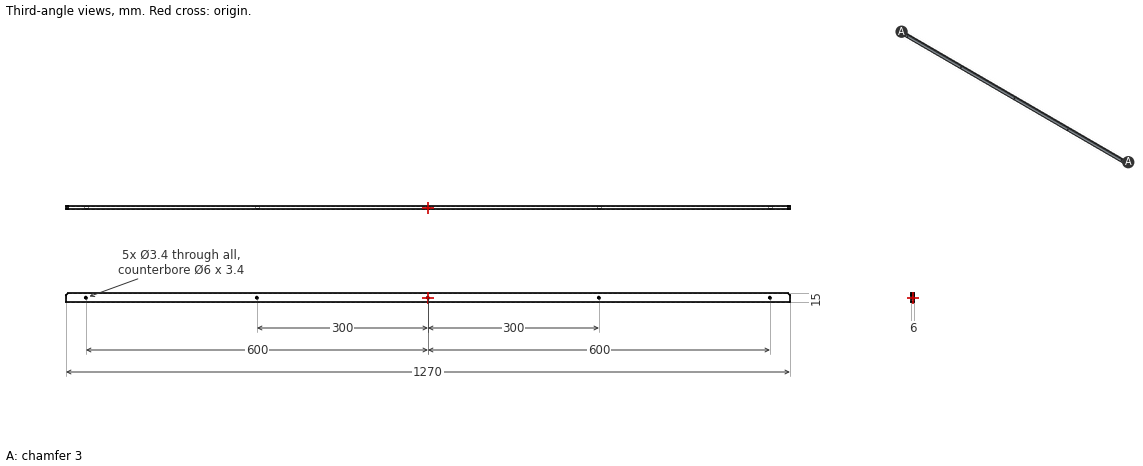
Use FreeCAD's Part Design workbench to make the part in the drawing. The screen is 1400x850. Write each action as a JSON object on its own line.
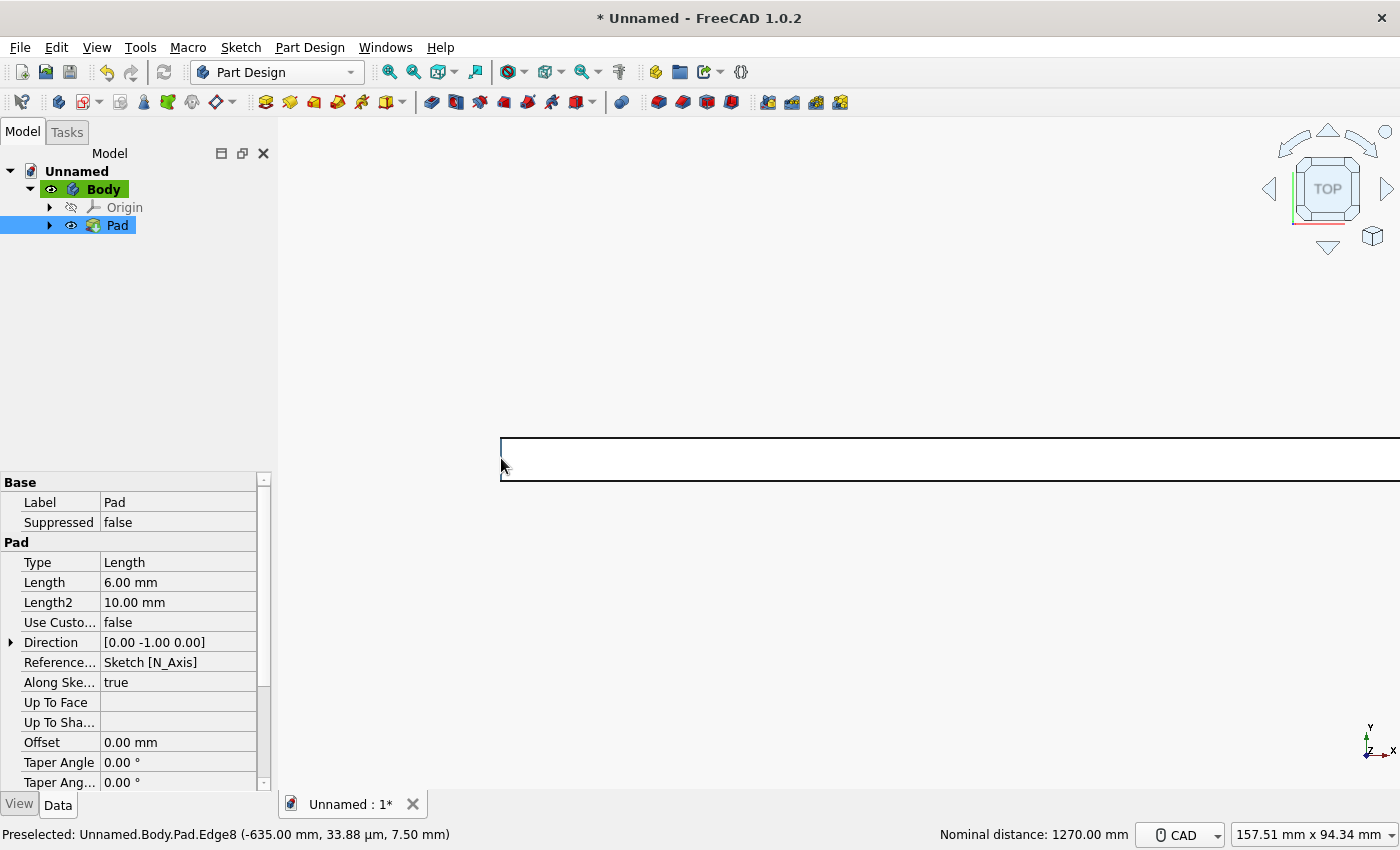
{"action": "left_click", "coordinate": [684, 102]}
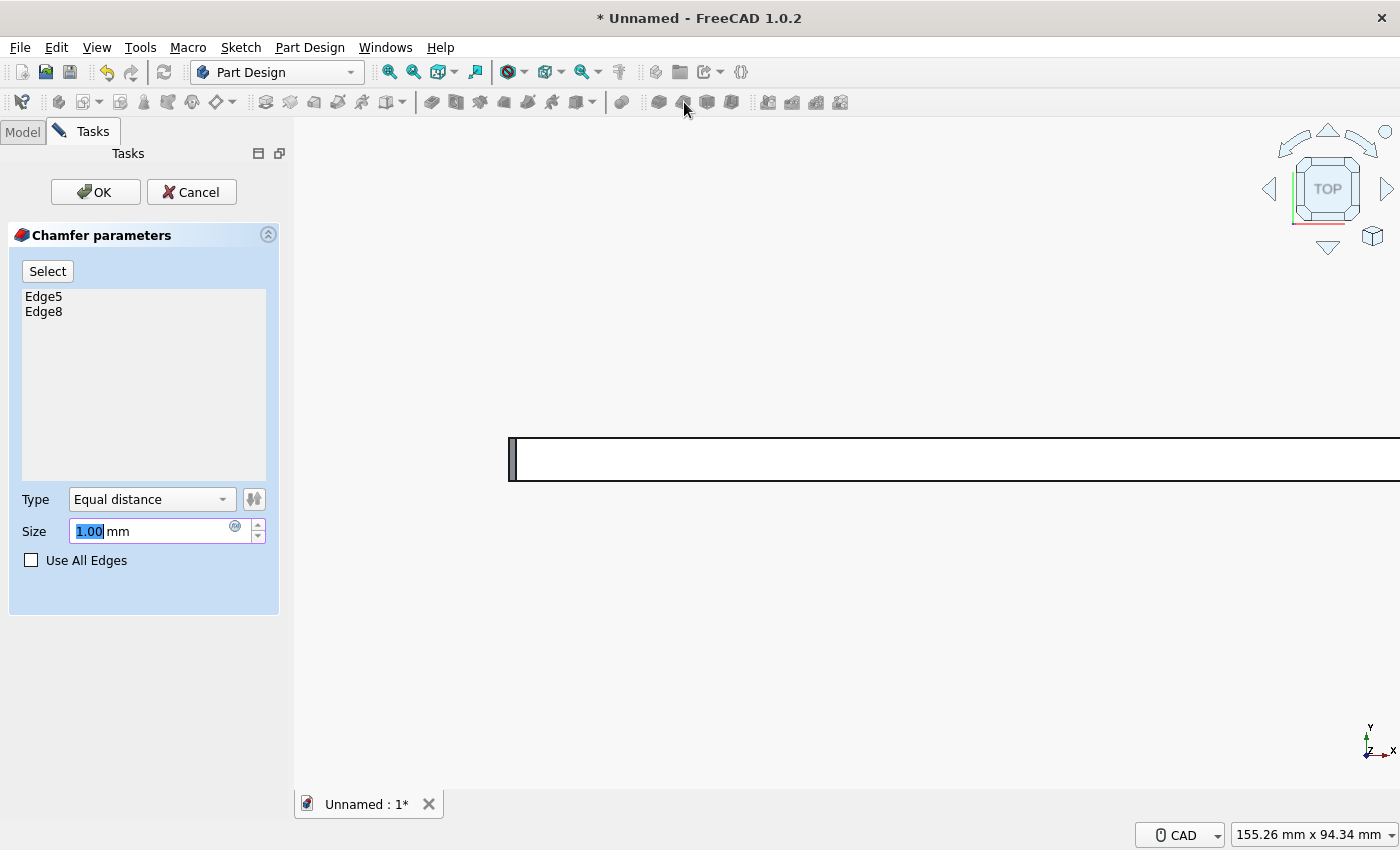
{"action": "type", "text": "3"}
{"action": "key", "text": "Tab"}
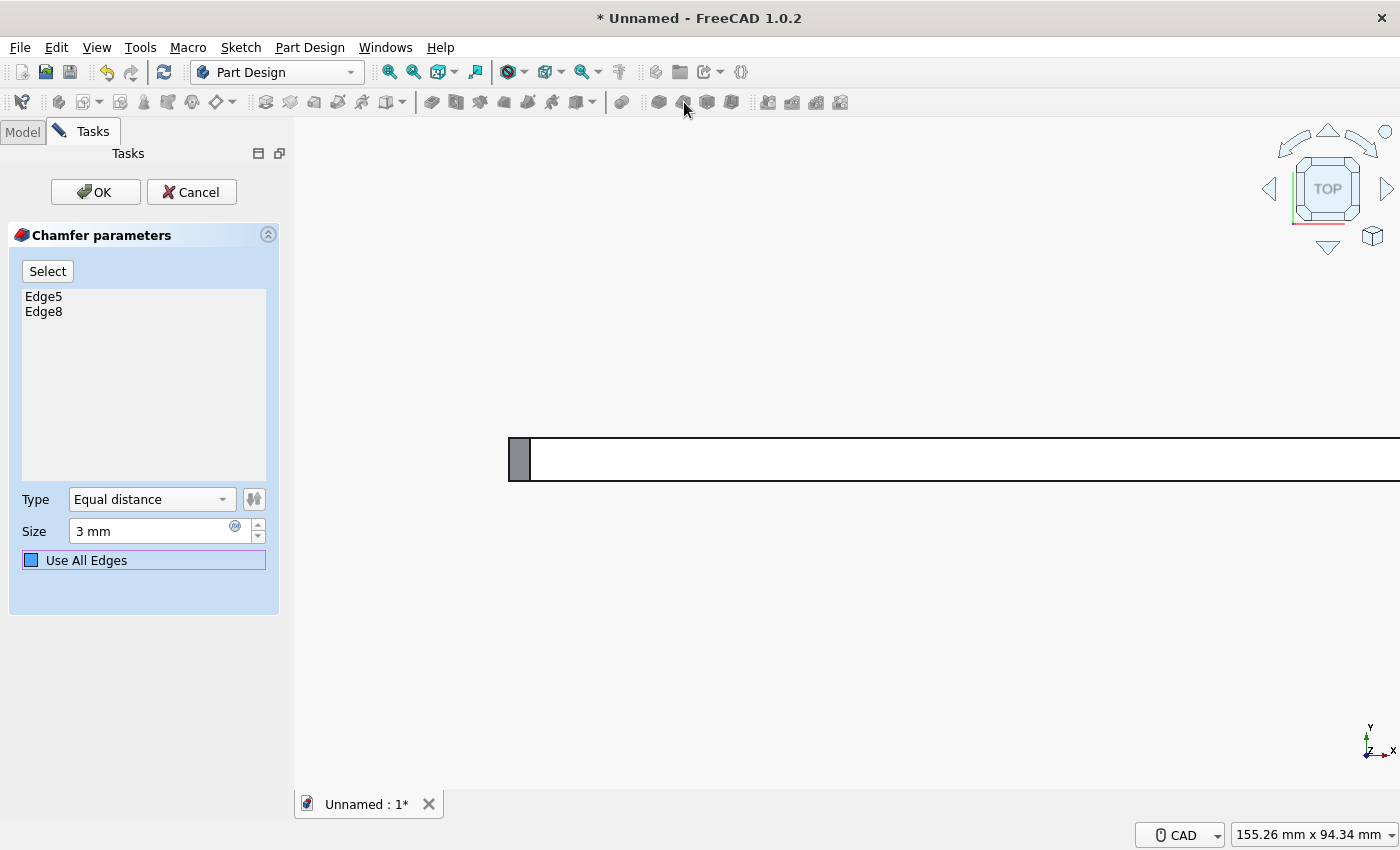
{"action": "left_click", "coordinate": [96, 192]}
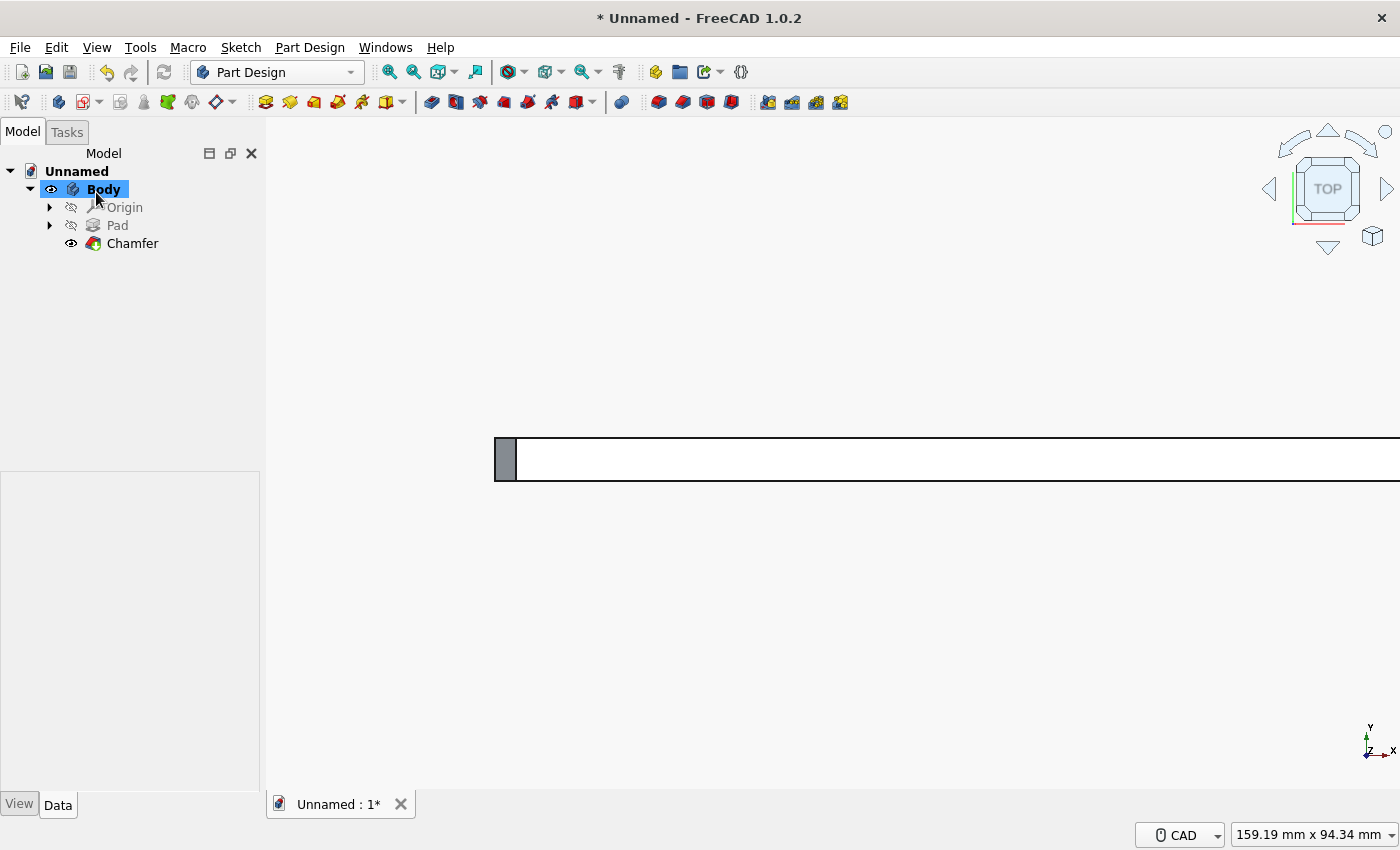
{"action": "left_click", "coordinate": [390, 72]}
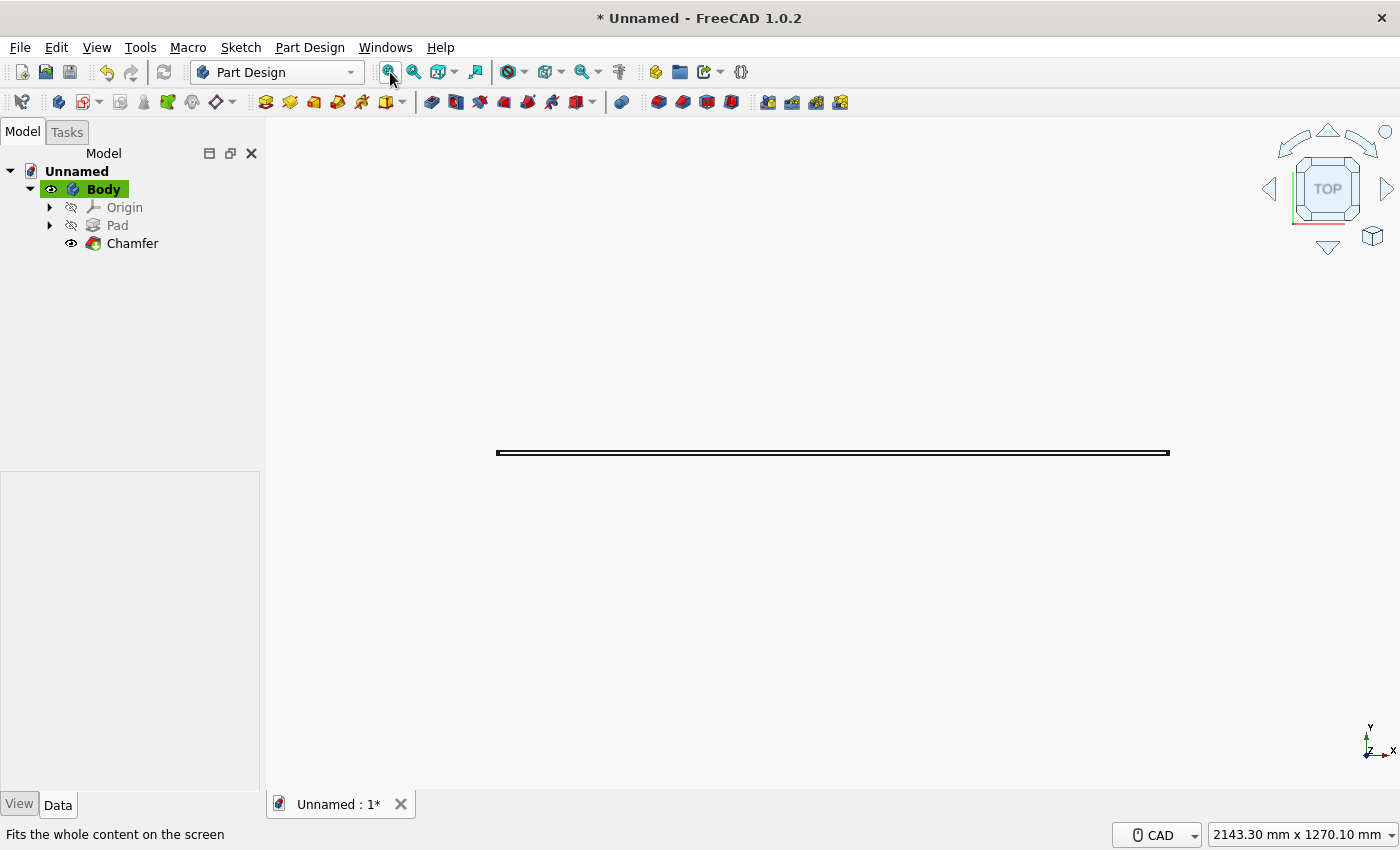
{"action": "key", "text": "4"}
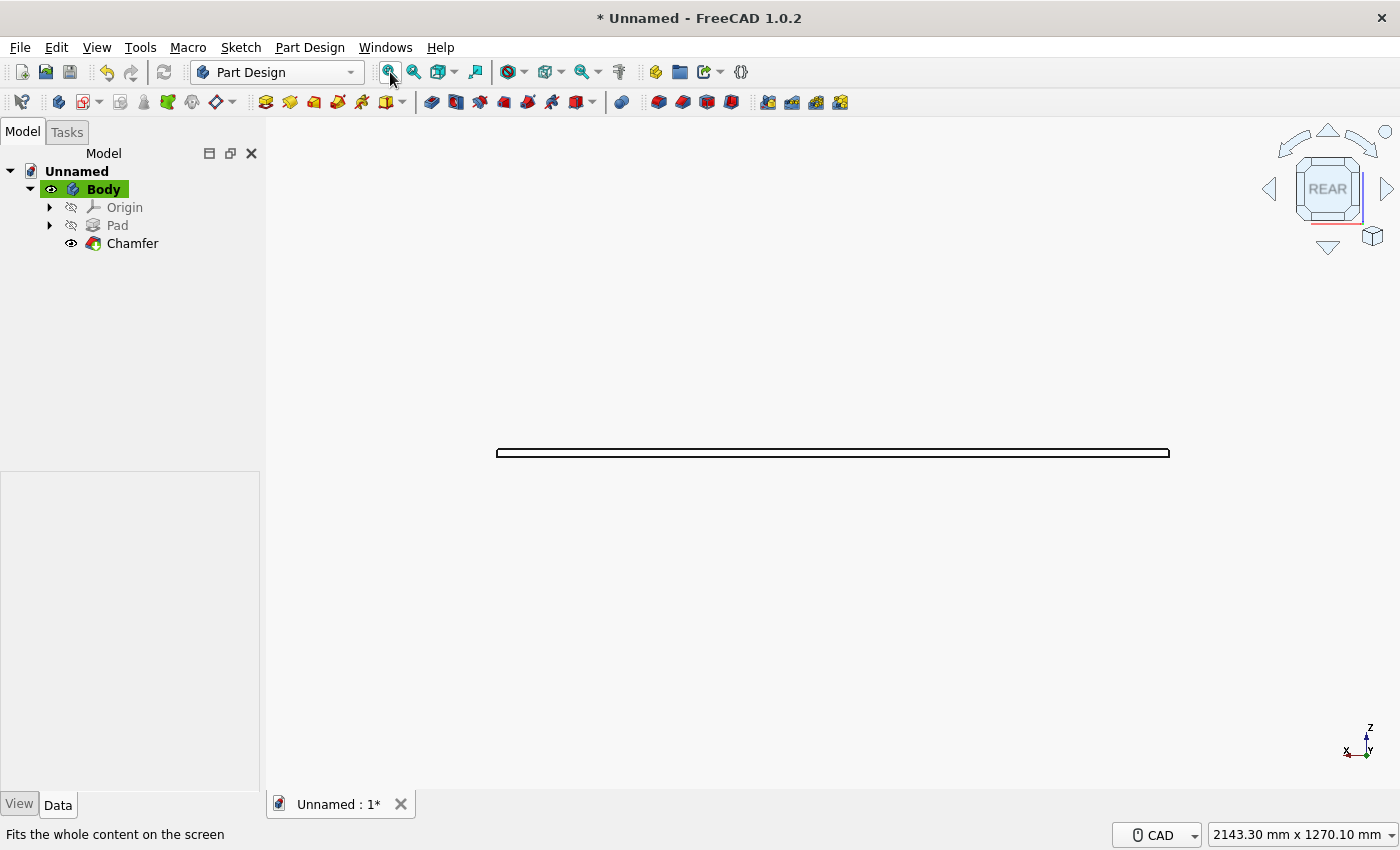
{"action": "scroll", "coordinate": [545, 452], "scroll_direction": "up", "scroll_amount": 6}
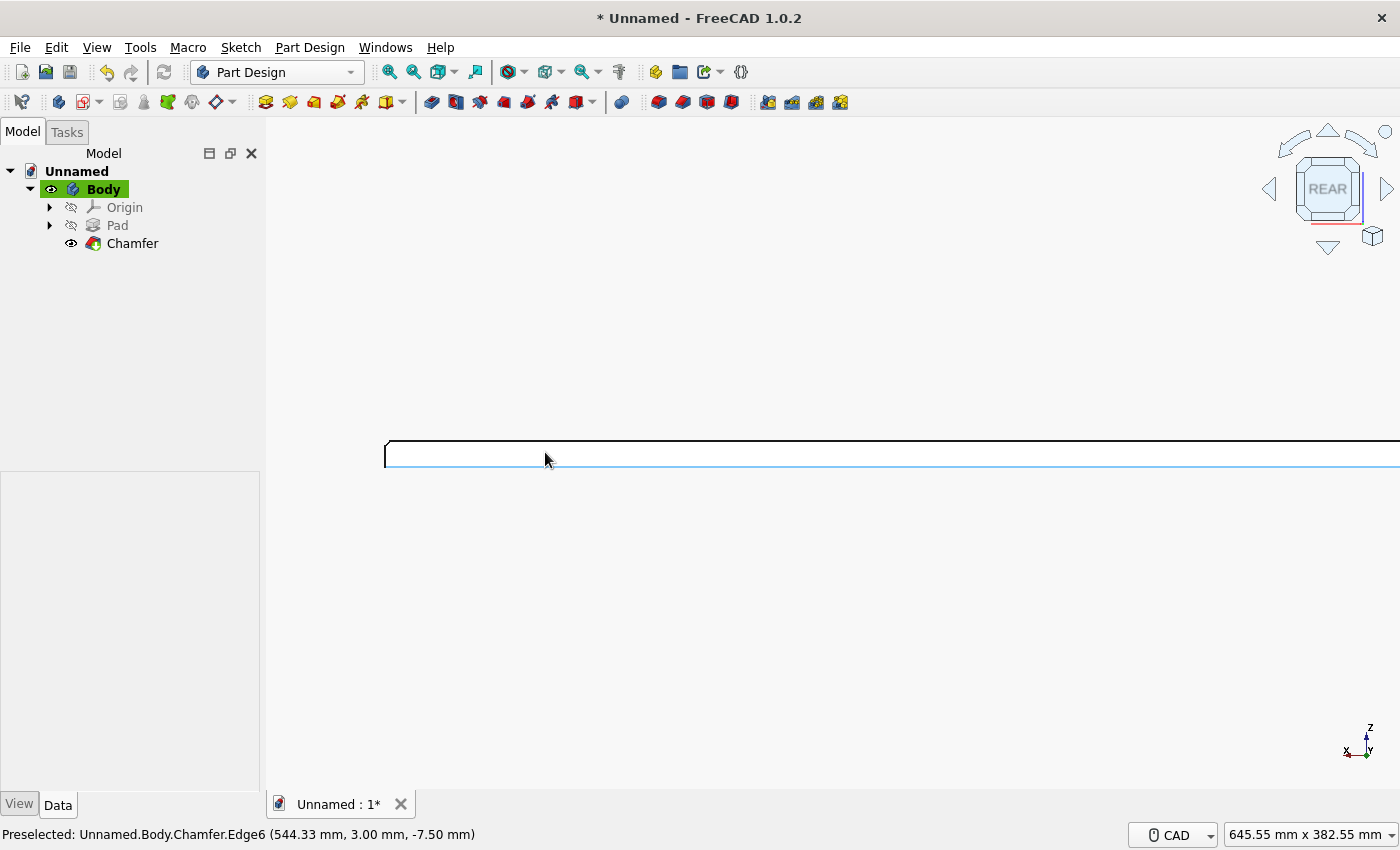
{"action": "left_click", "coordinate": [545, 453]}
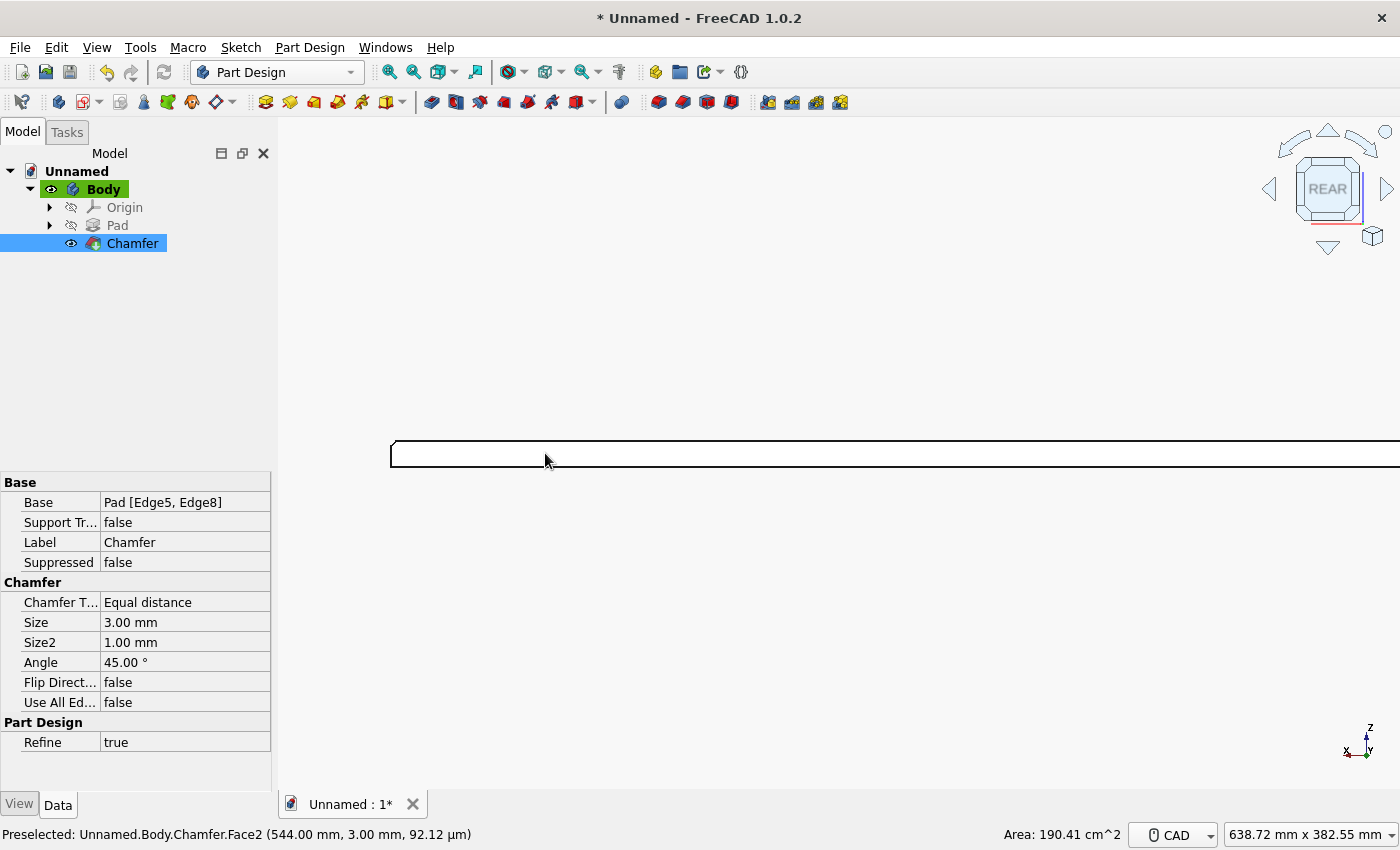
{"action": "left_click", "coordinate": [84, 102]}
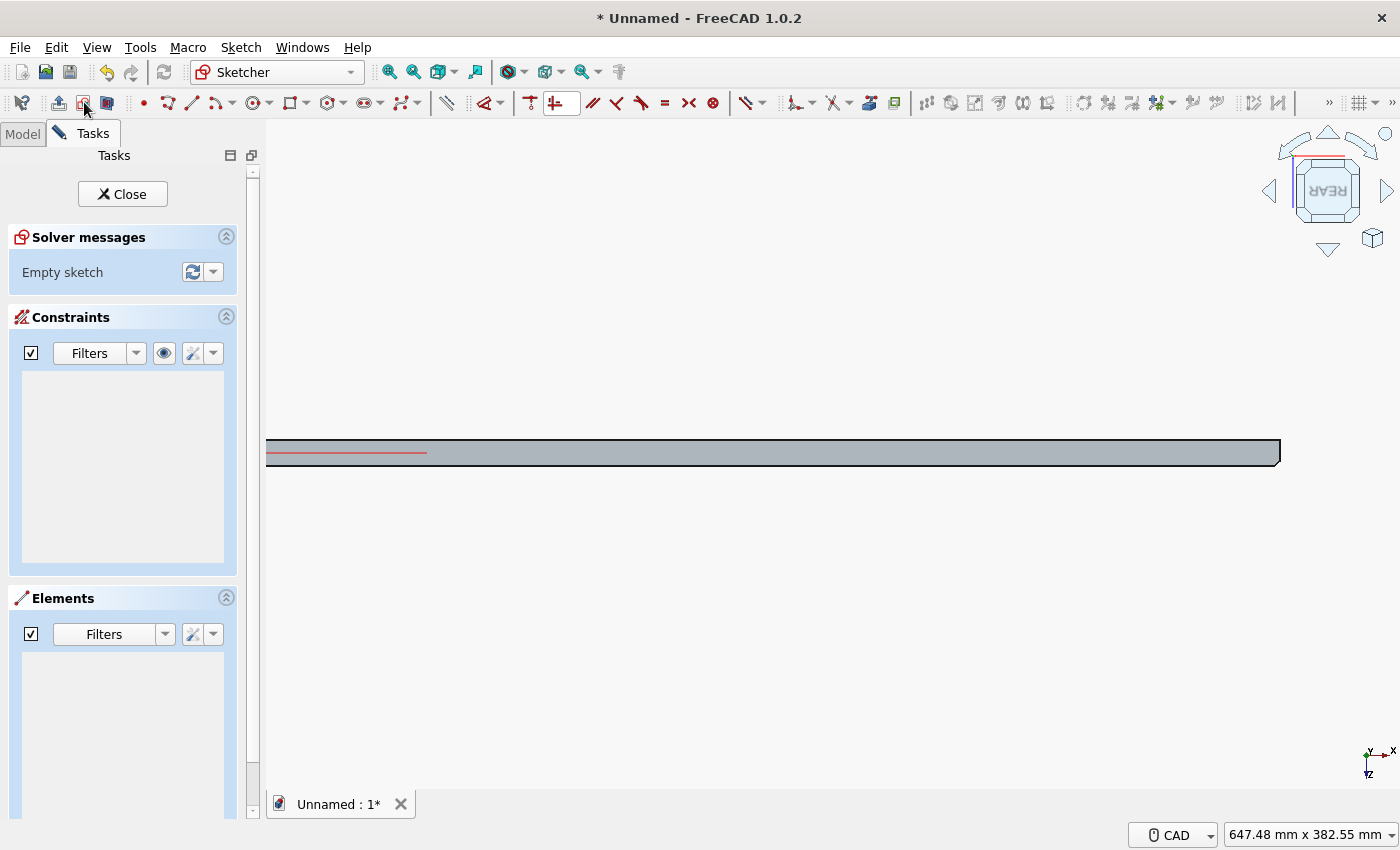
{"action": "scroll", "coordinate": [1022, 454], "scroll_direction": "down", "scroll_amount": 6}